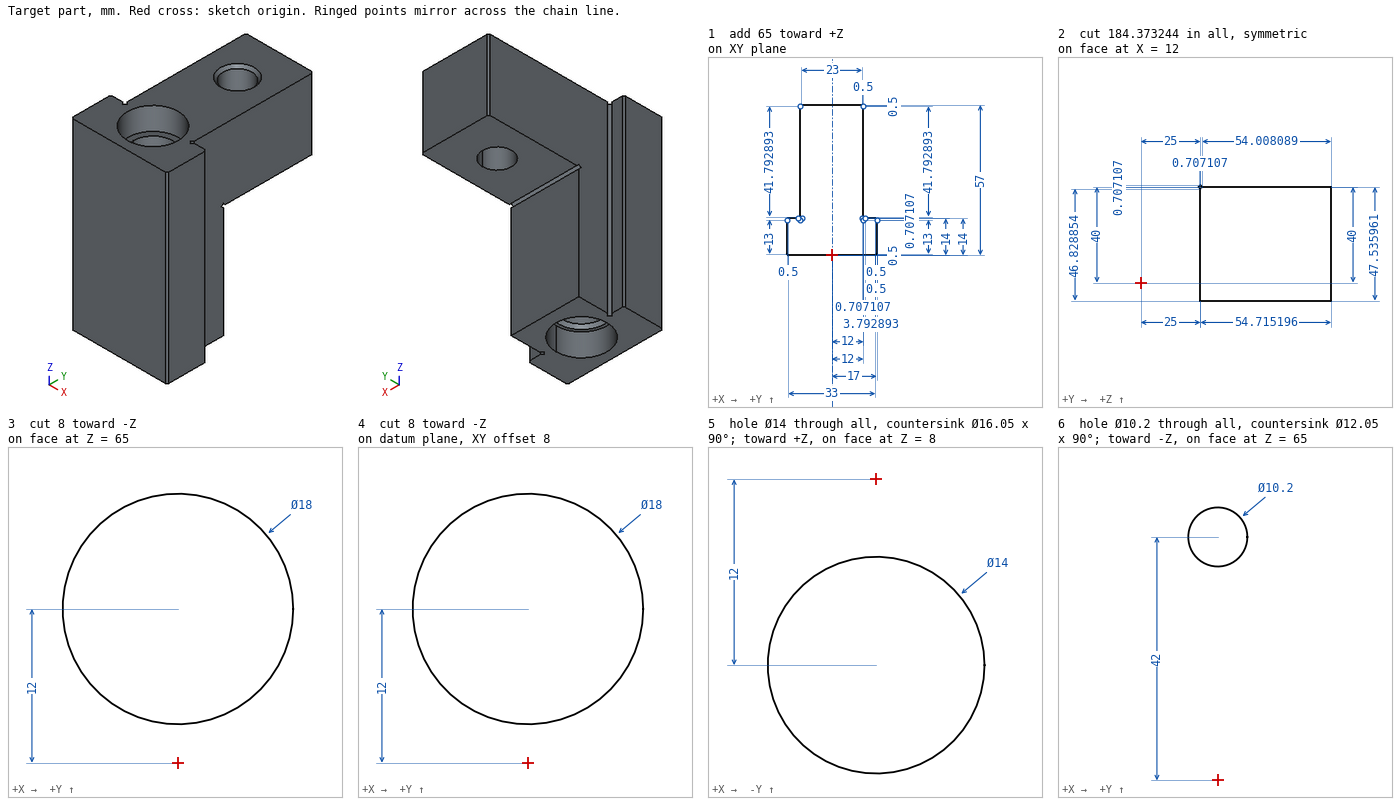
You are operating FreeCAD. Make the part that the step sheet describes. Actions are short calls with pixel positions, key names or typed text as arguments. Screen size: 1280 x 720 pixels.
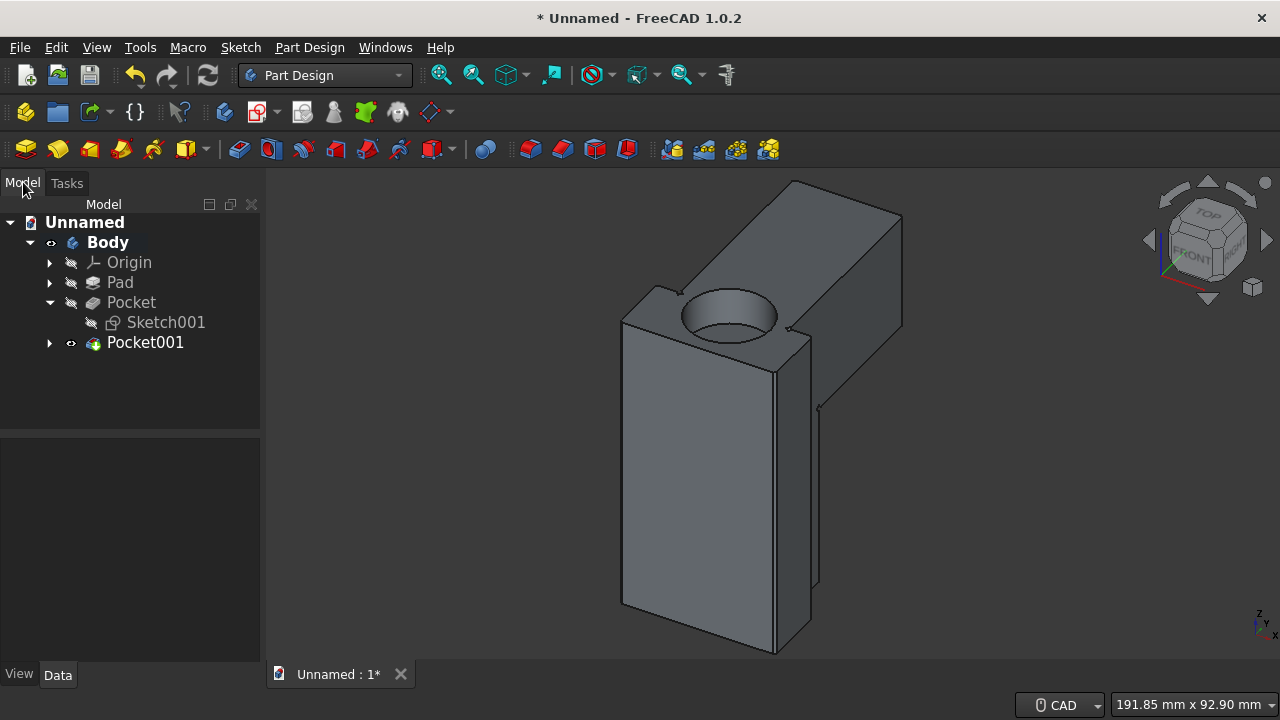
click(50, 263)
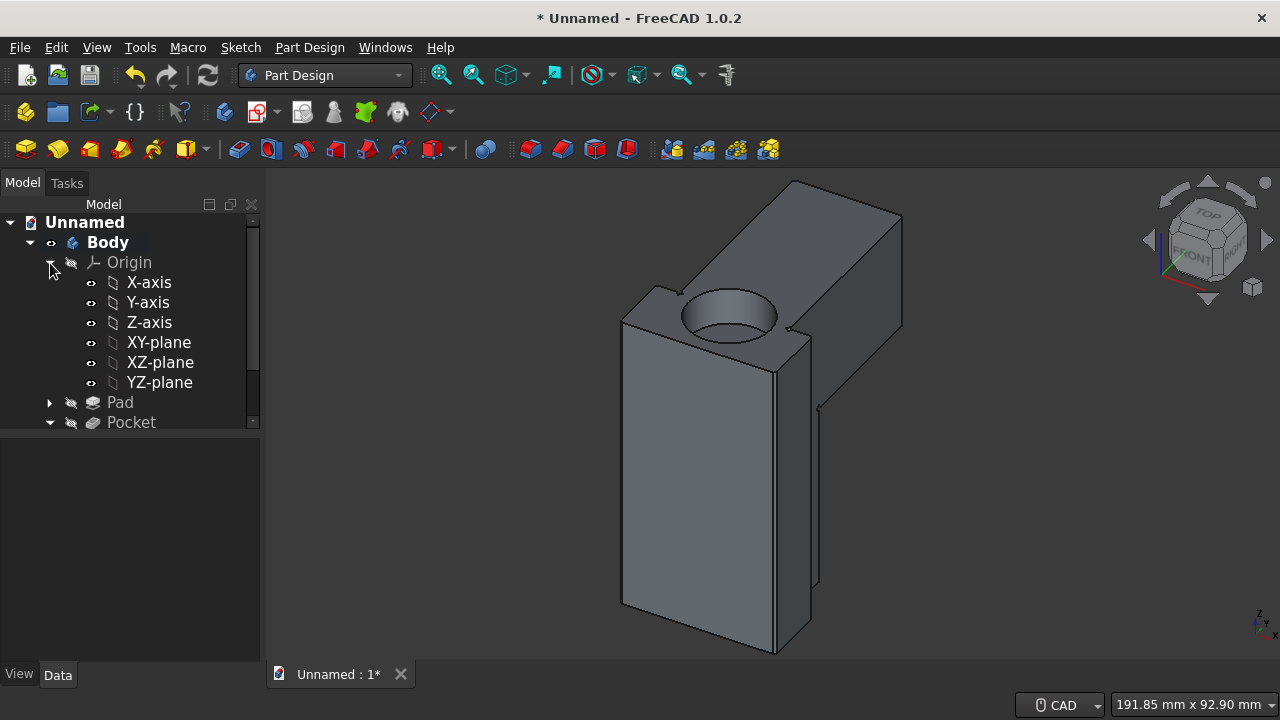
click(136, 343)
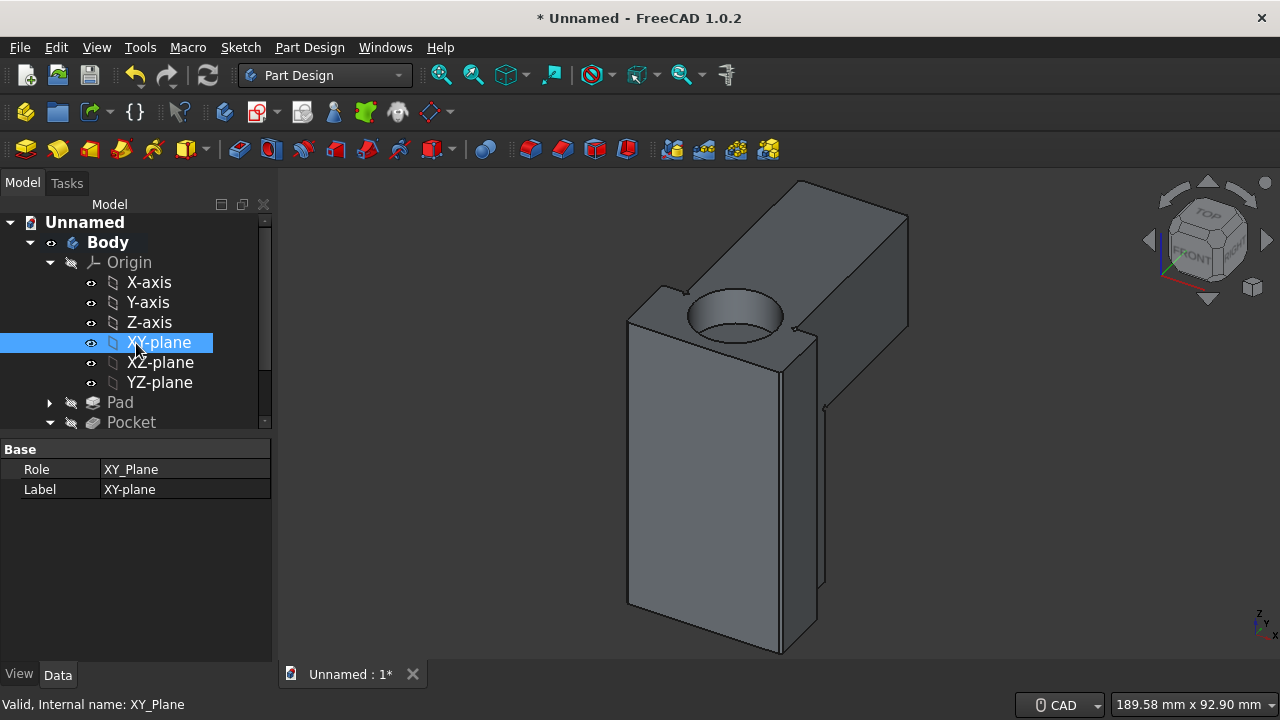
click(430, 112)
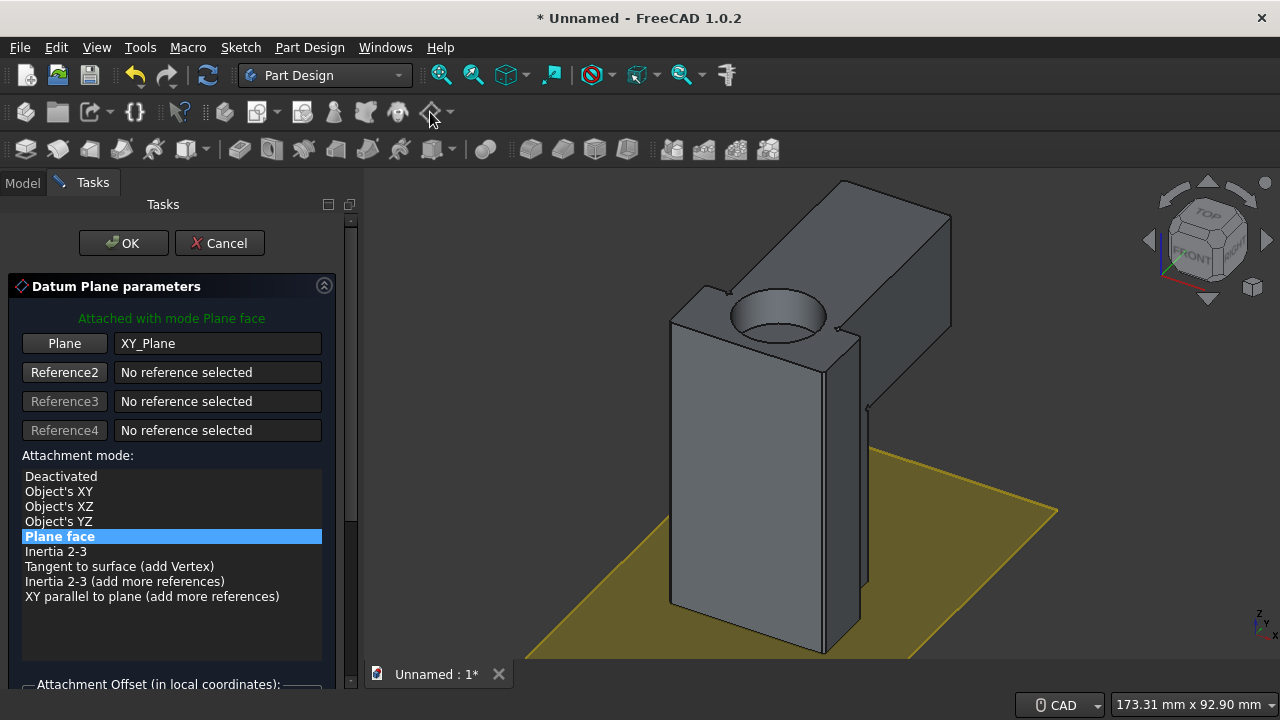
scroll(351, 451, down, 3)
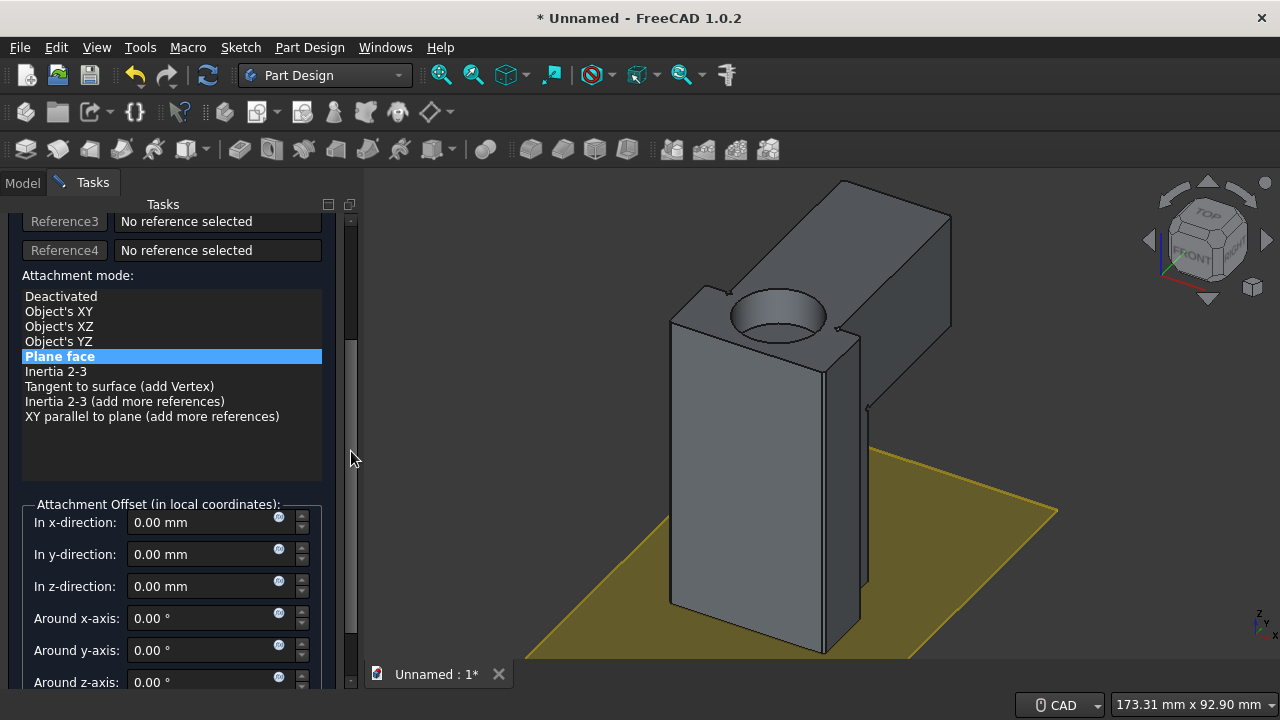
triple_click(210, 586)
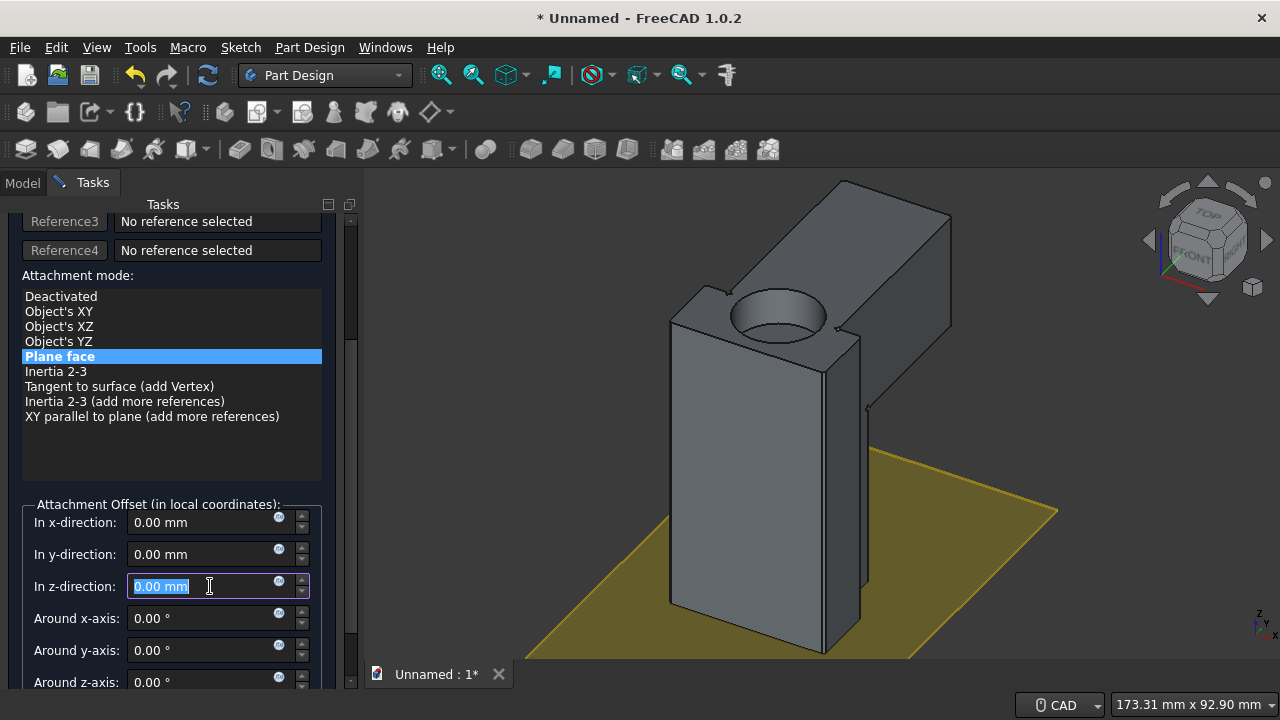
text(8)
key(Tab)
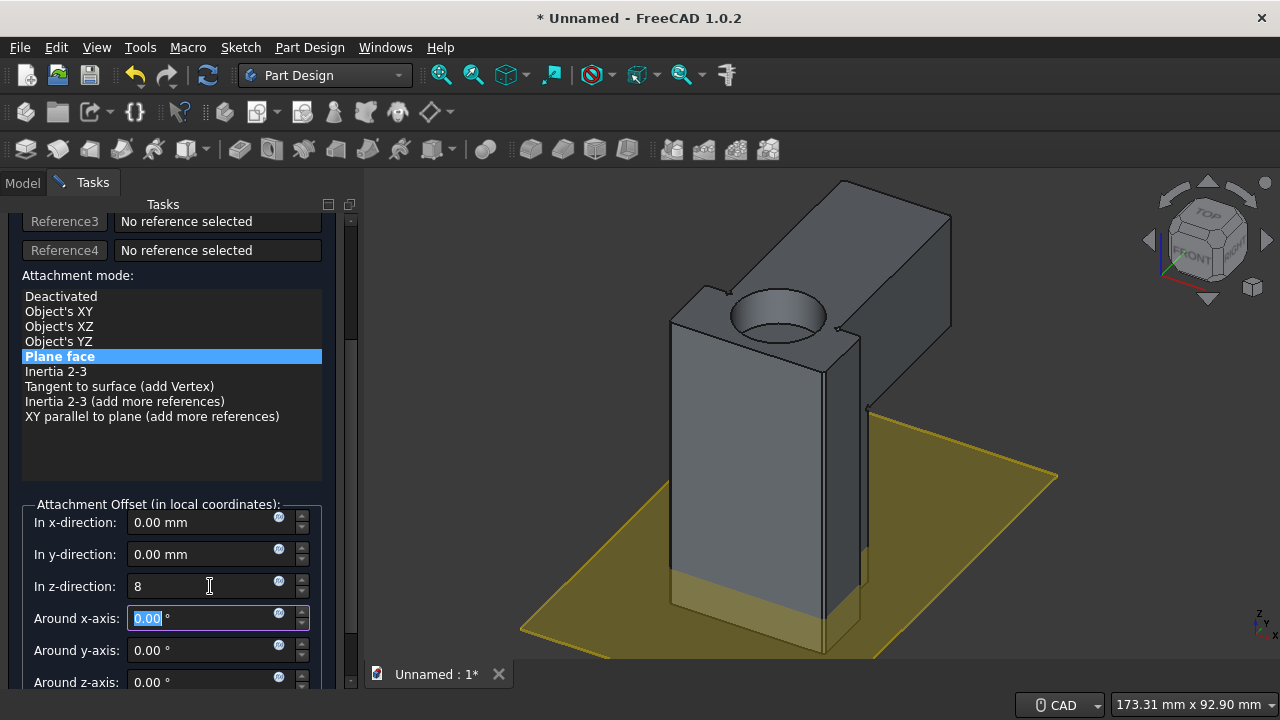
scroll(351, 451, up, 4)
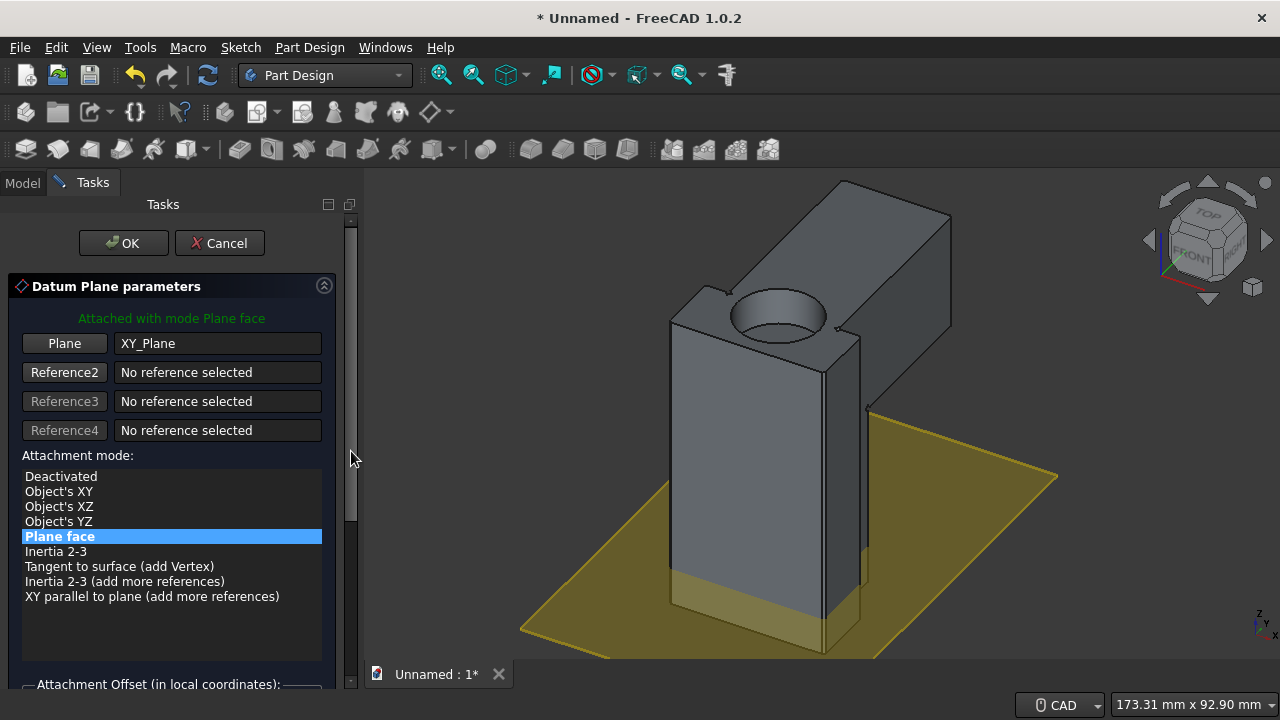
click(124, 243)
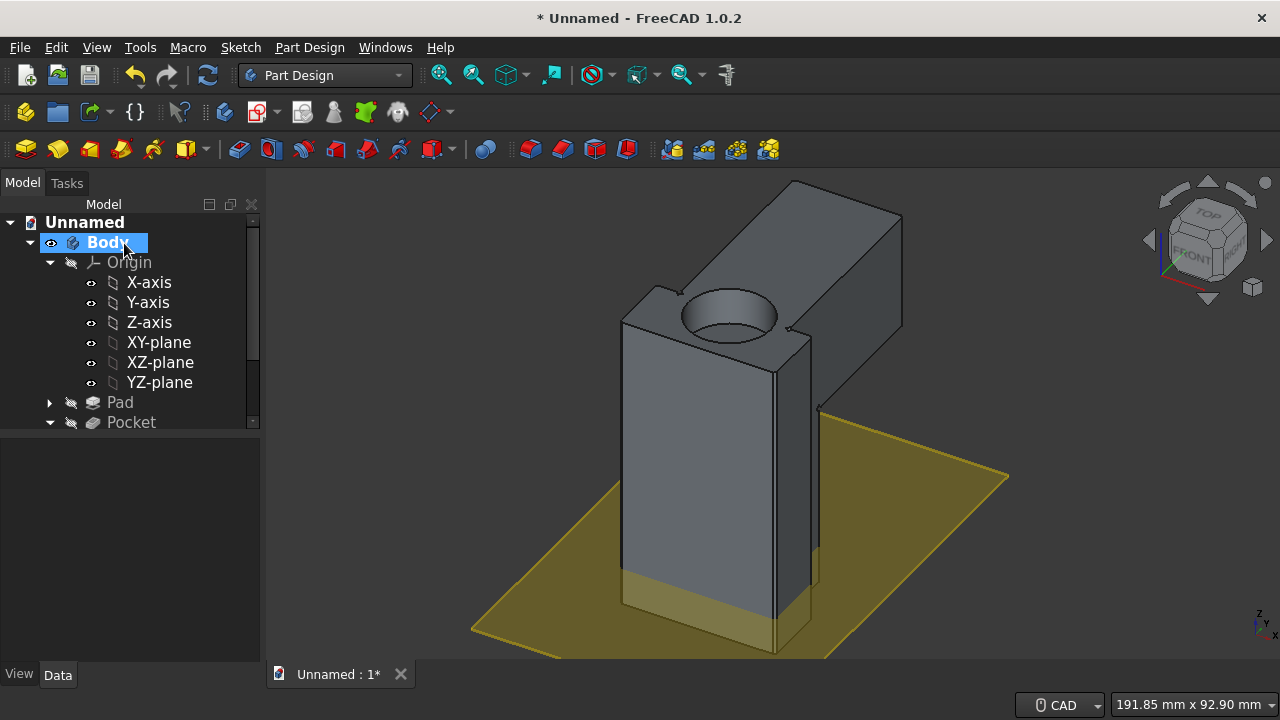
scroll(100, 318, down, 3)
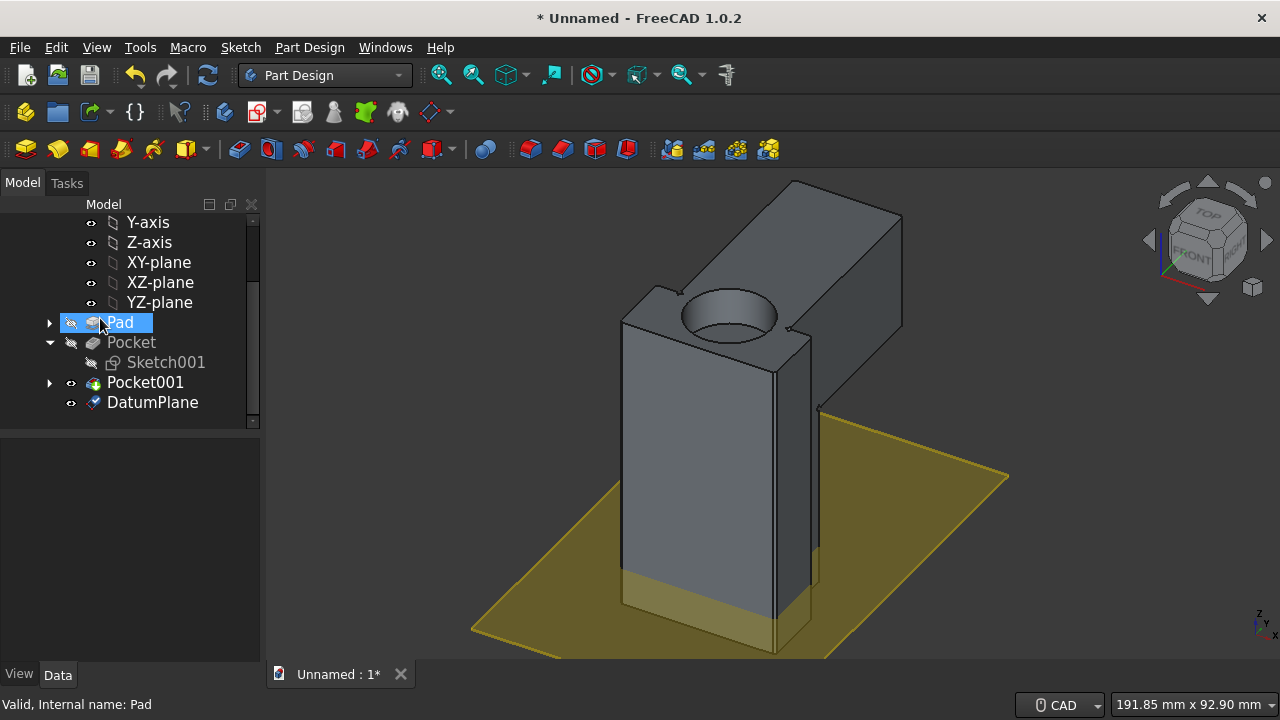
click(116, 403)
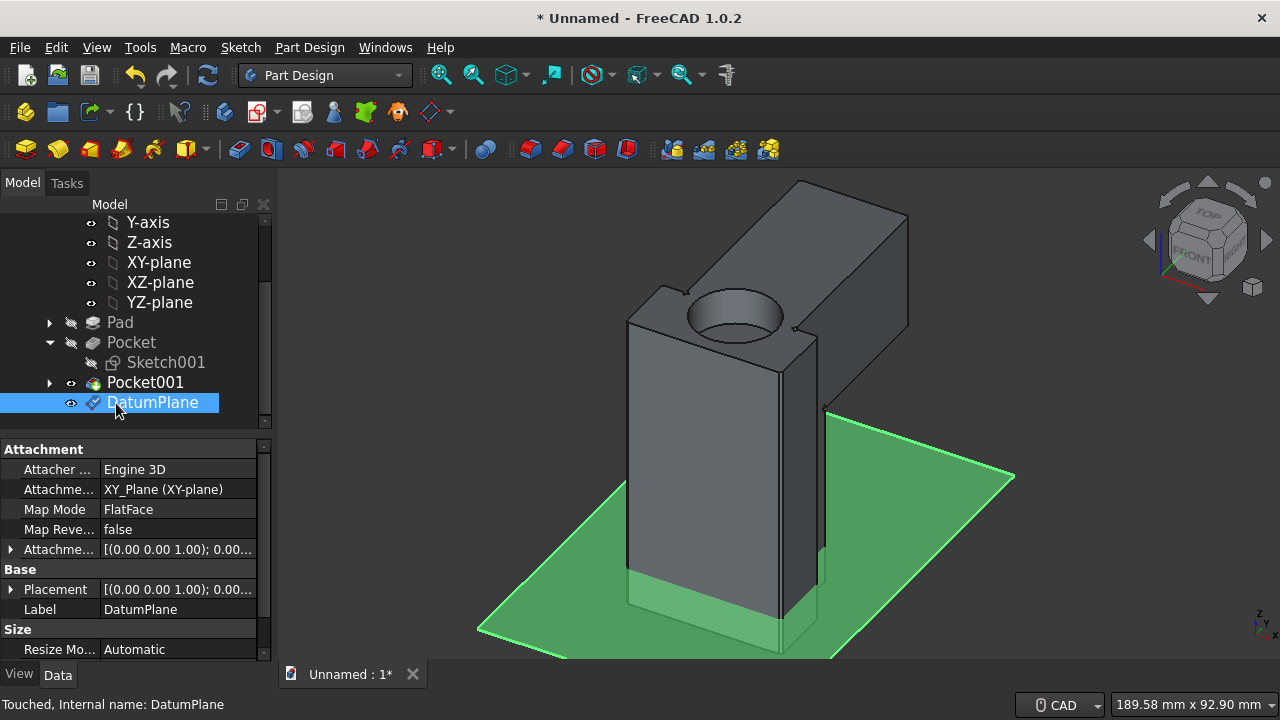
click(258, 112)